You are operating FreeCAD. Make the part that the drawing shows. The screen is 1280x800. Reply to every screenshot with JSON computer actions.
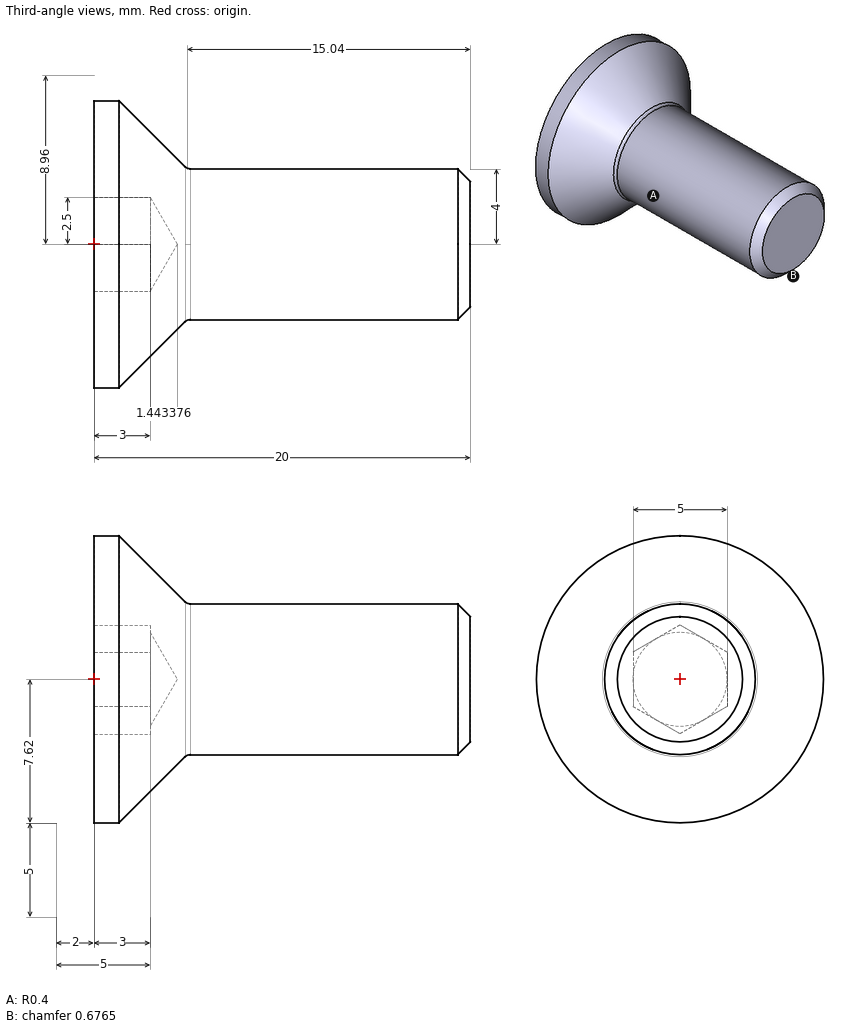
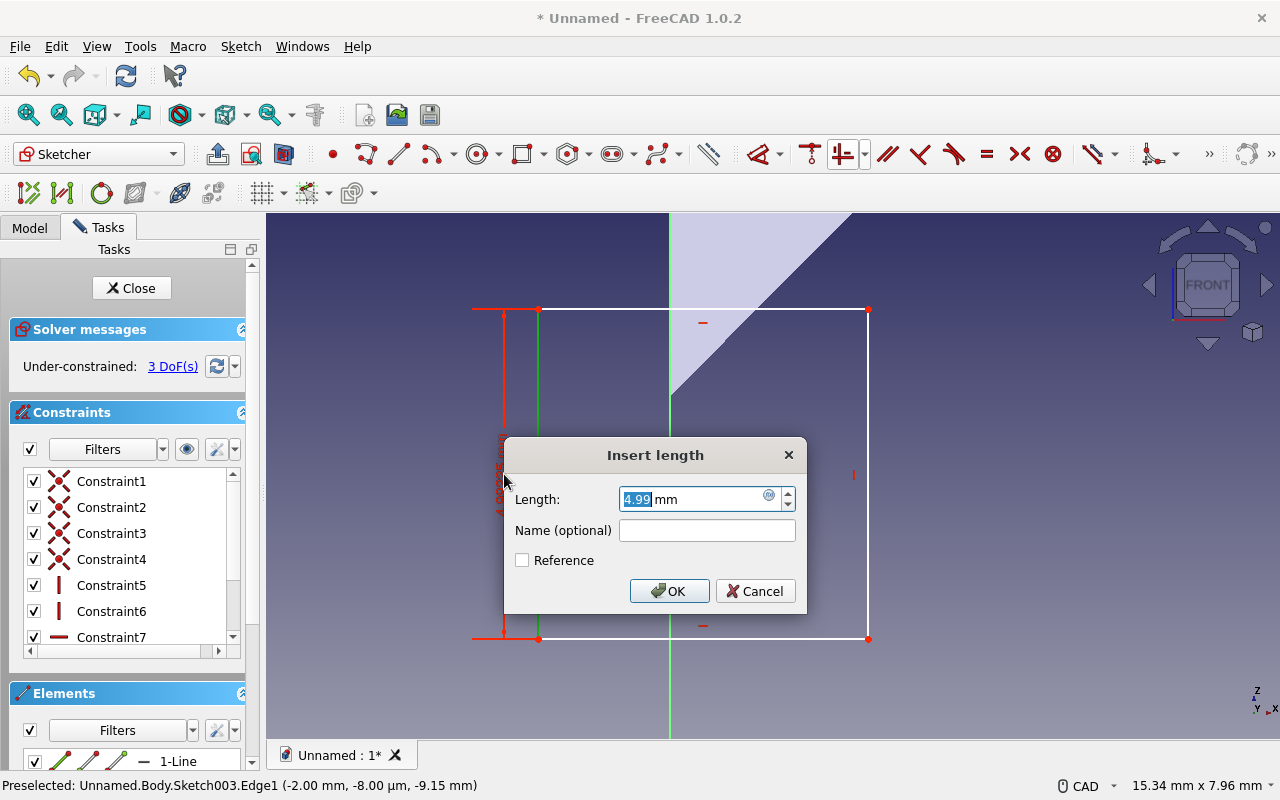
{"action": "type", "text": "5"}
{"action": "key", "text": "Return"}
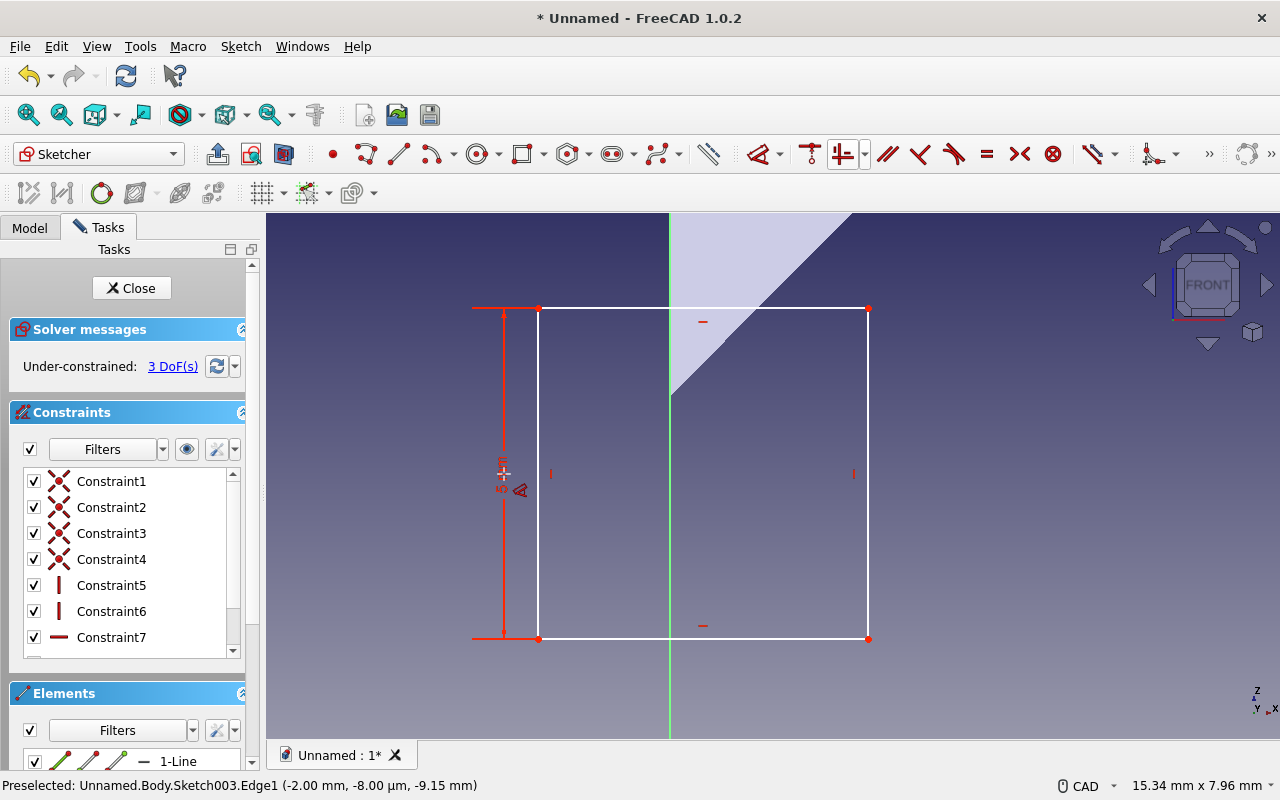
{"action": "left_click", "coordinate": [637, 639]}
{"action": "left_click", "coordinate": [703, 673]}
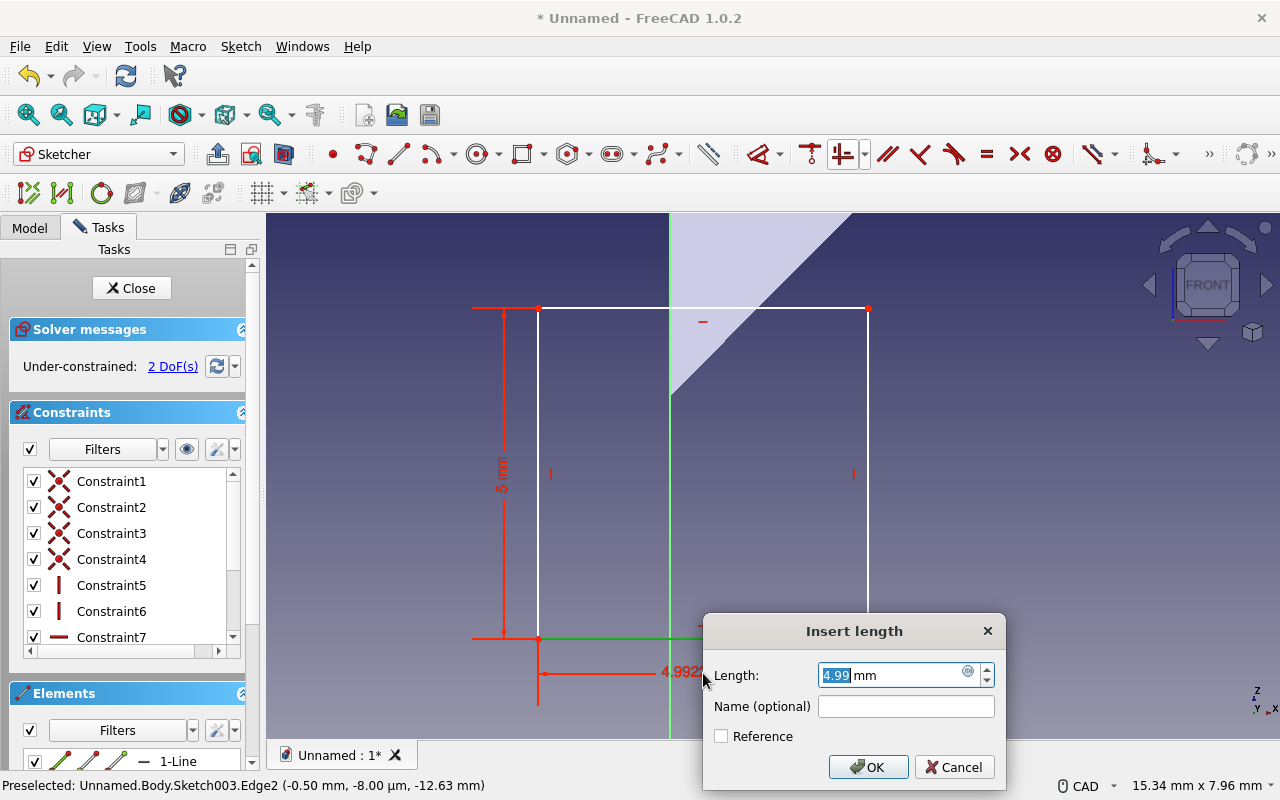
{"action": "type", "text": "5"}
{"action": "key", "text": "Return"}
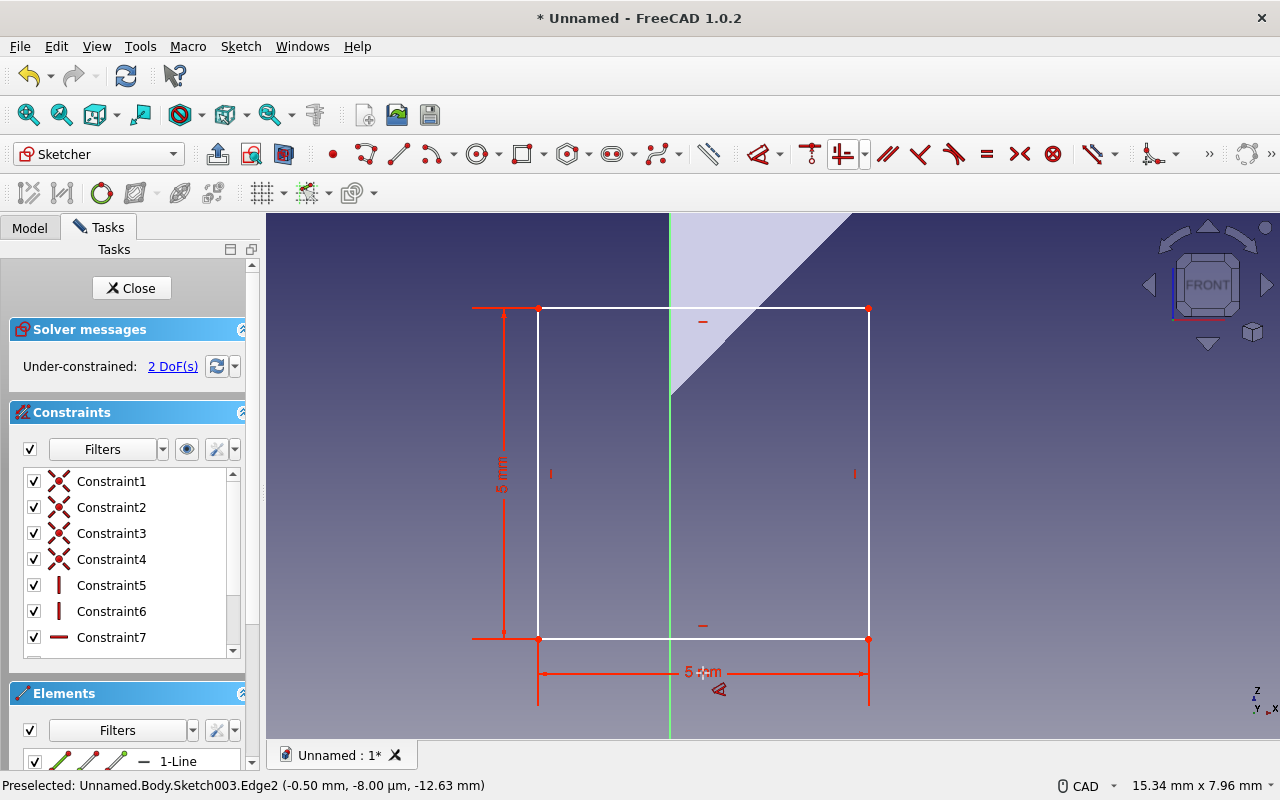
{"action": "left_click", "coordinate": [538, 308]}
{"action": "left_click", "coordinate": [604, 342]}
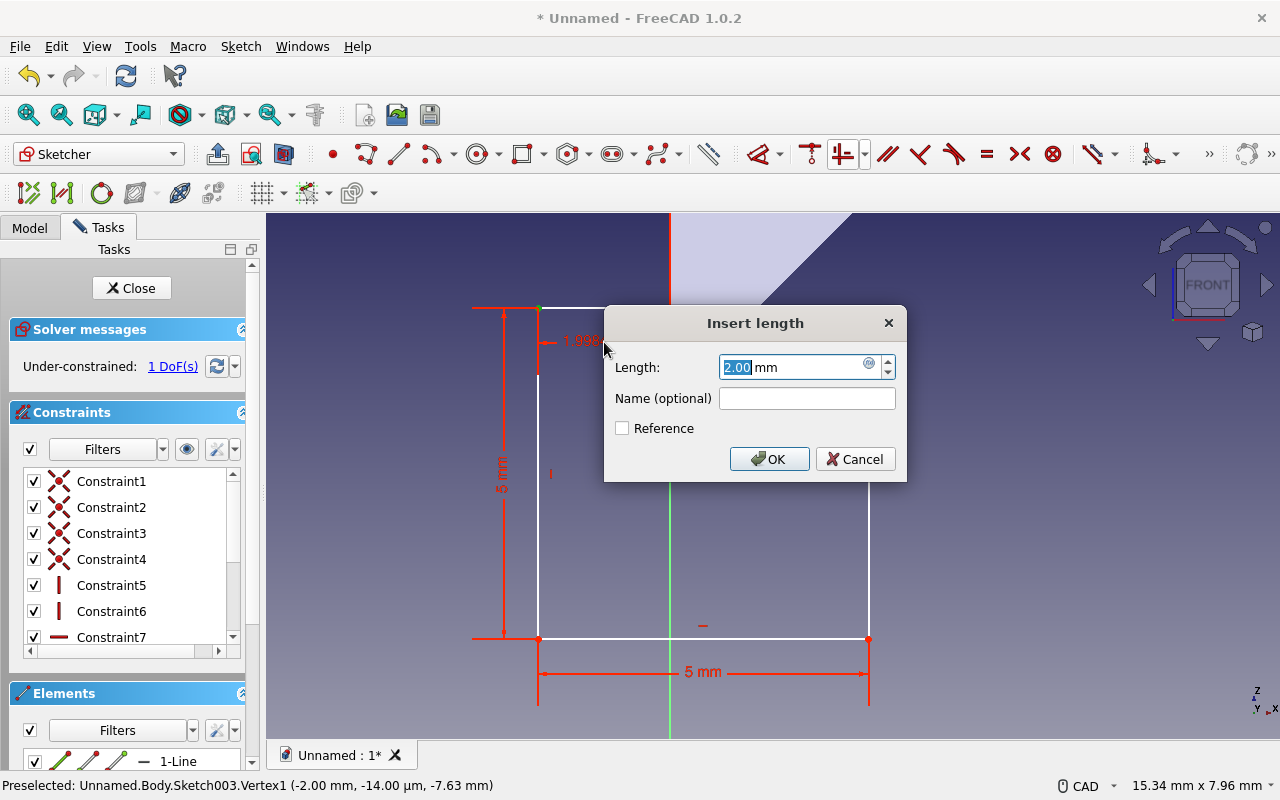
{"action": "type", "text": "2"}
{"action": "key", "text": "Return"}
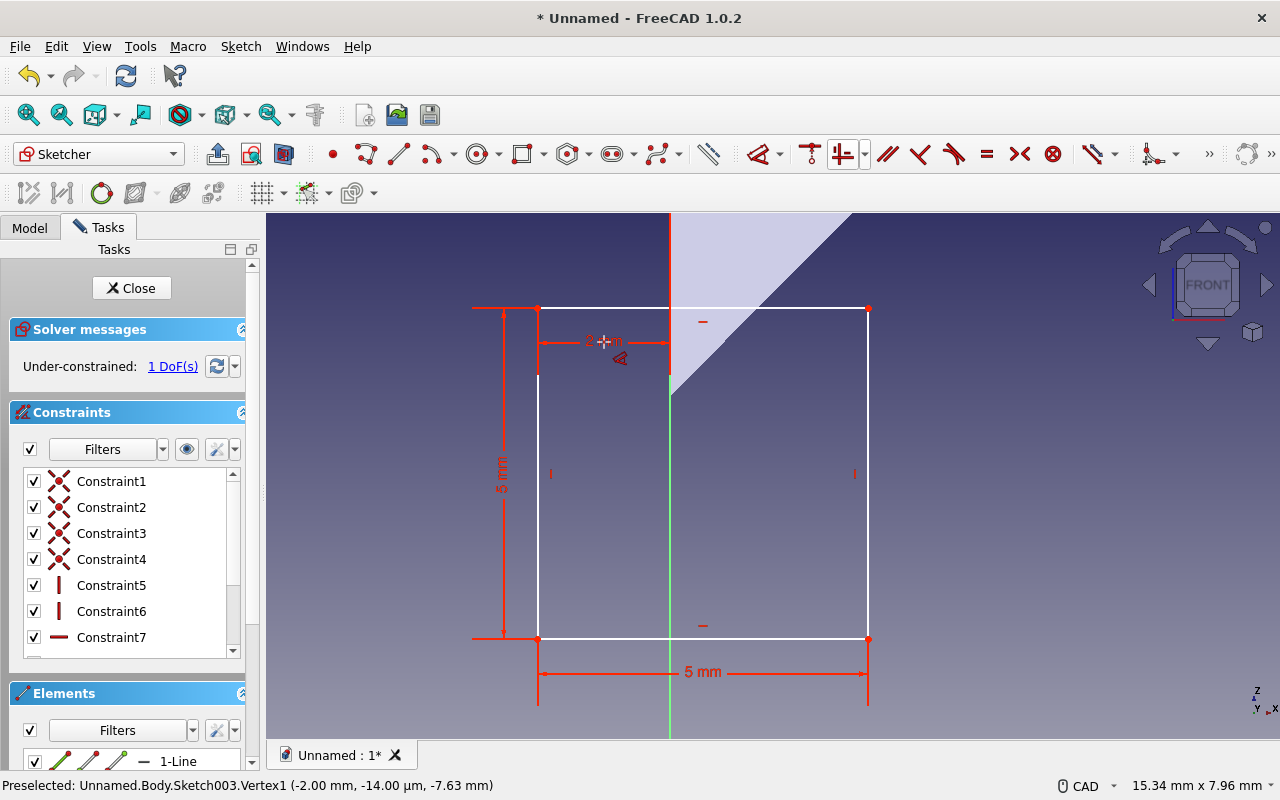
{"action": "left_click", "coordinate": [538, 308]}
{"action": "left_click", "coordinate": [504, 275]}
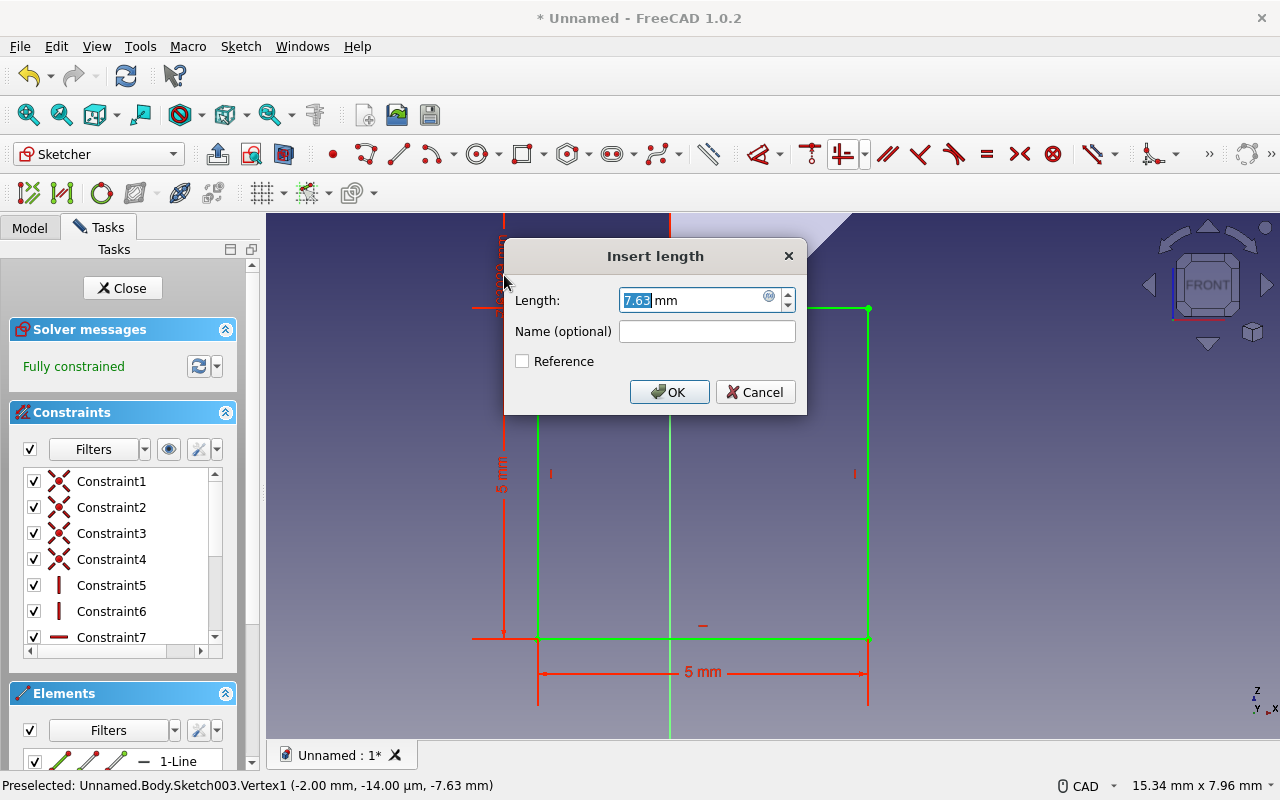
{"action": "type", "text": "7.62"}
{"action": "key", "text": "Return"}
{"action": "key", "text": "Escape"}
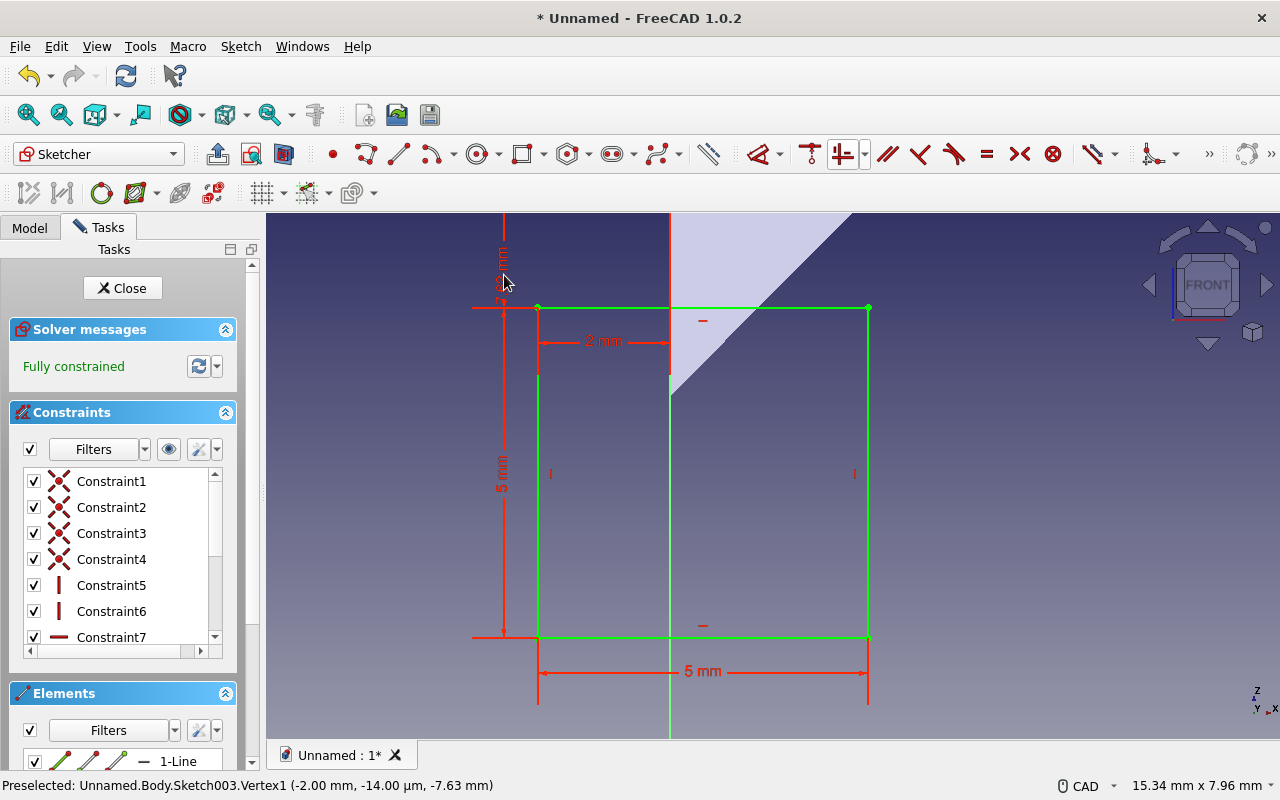
{"action": "left_click", "coordinate": [123, 288]}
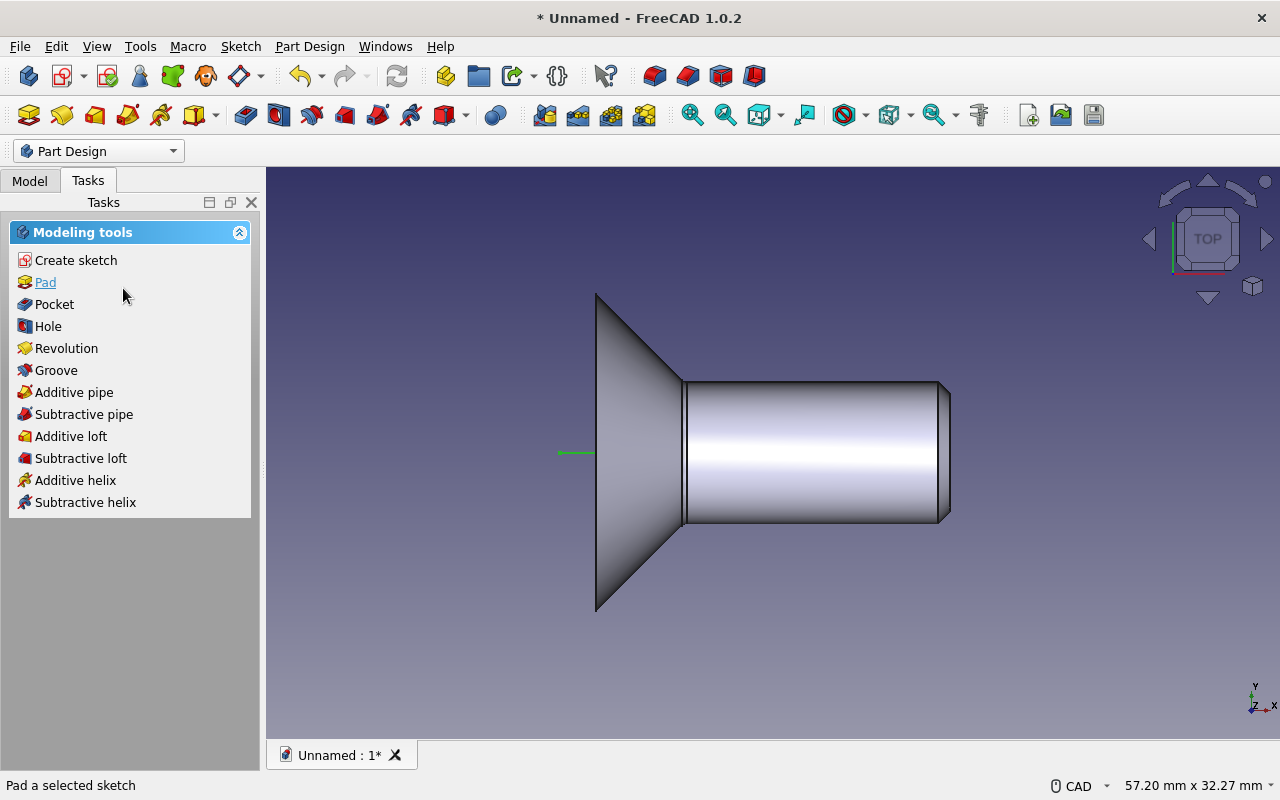
{"action": "left_click", "coordinate": [312, 116]}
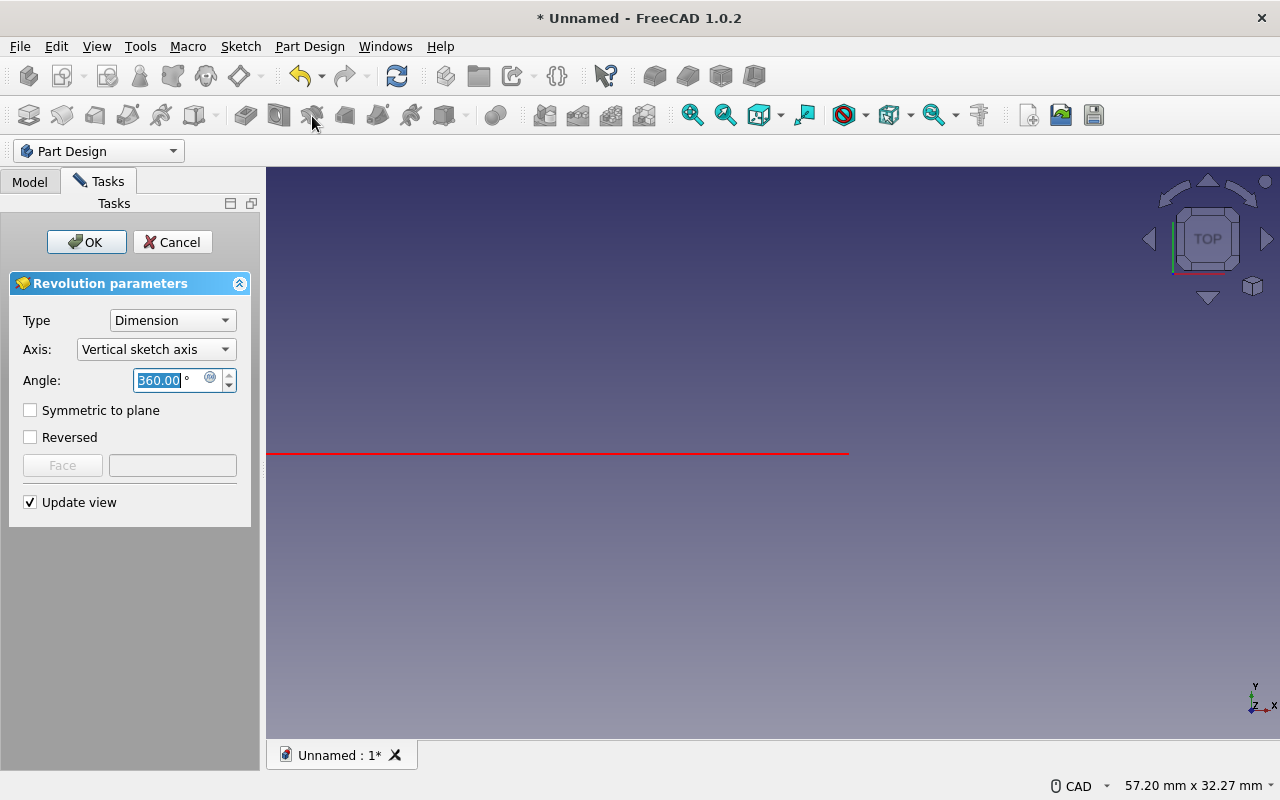
{"action": "left_click", "coordinate": [157, 350]}